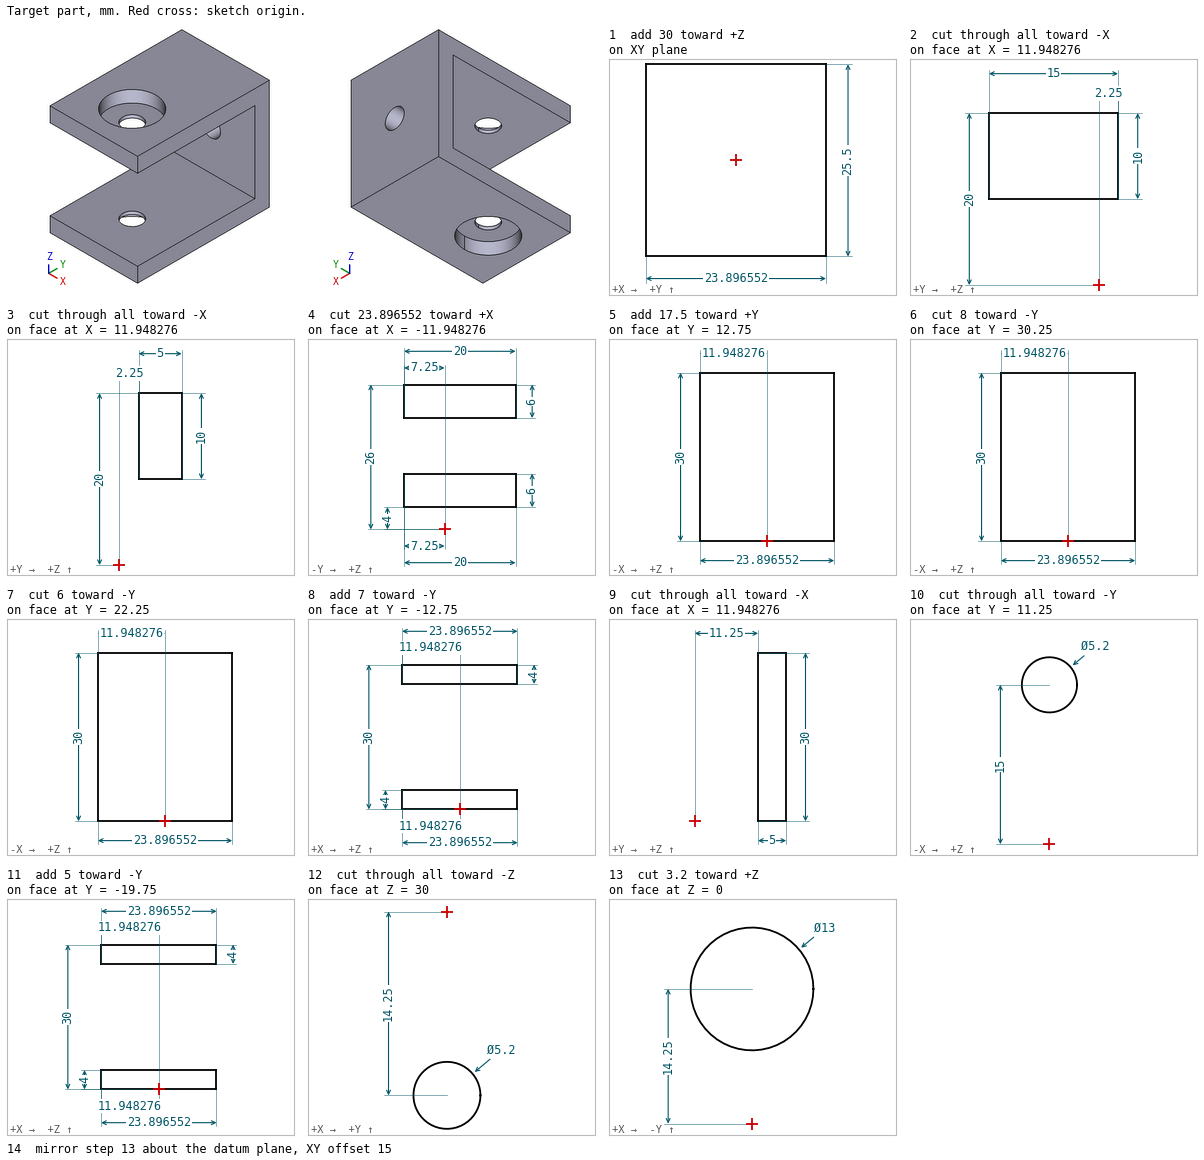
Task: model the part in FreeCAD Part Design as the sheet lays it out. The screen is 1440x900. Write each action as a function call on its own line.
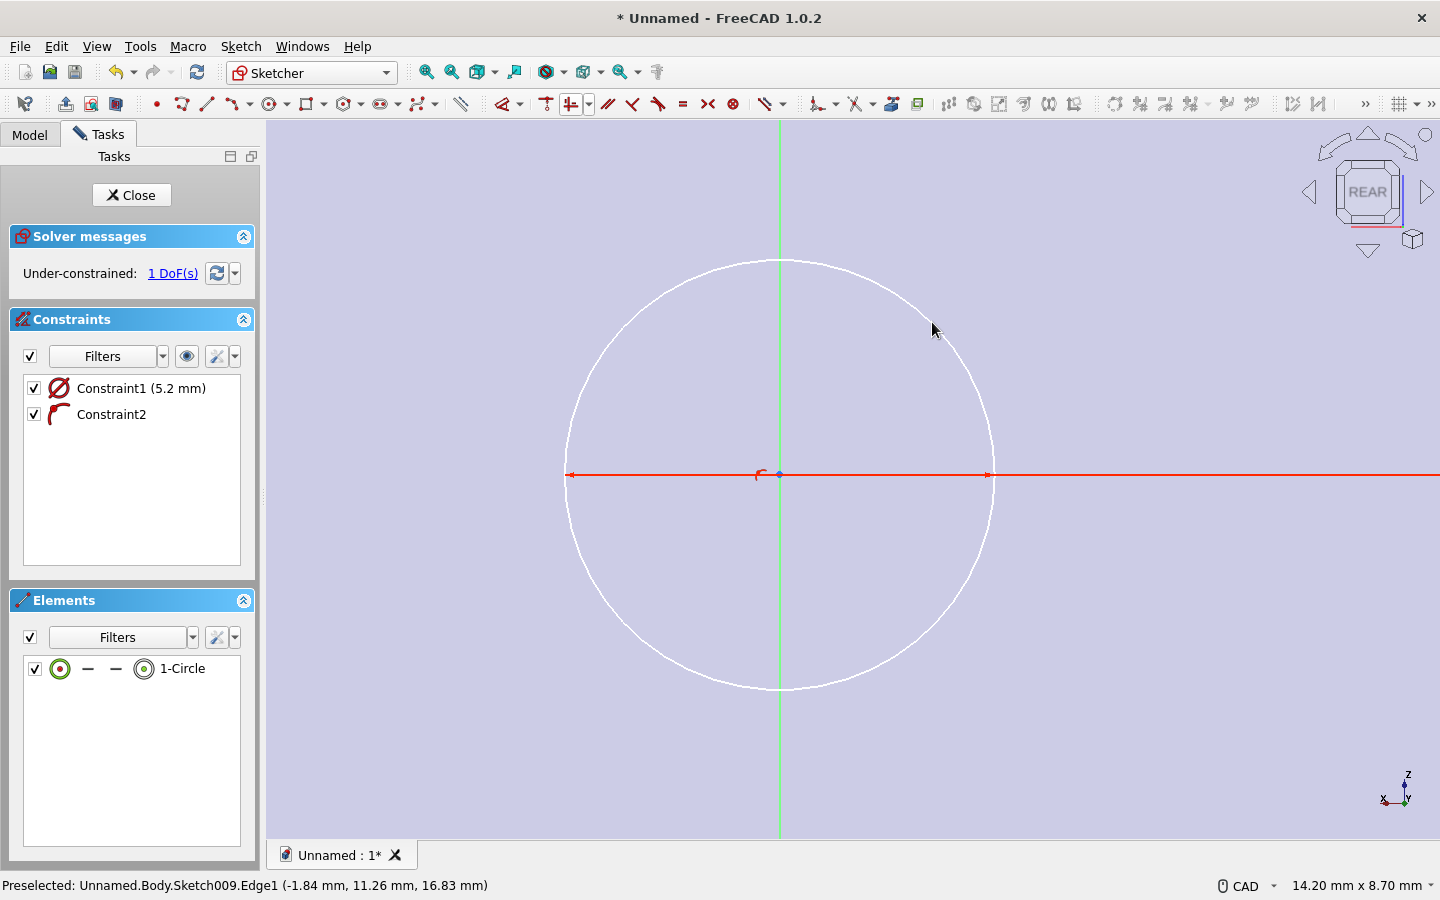
key(d)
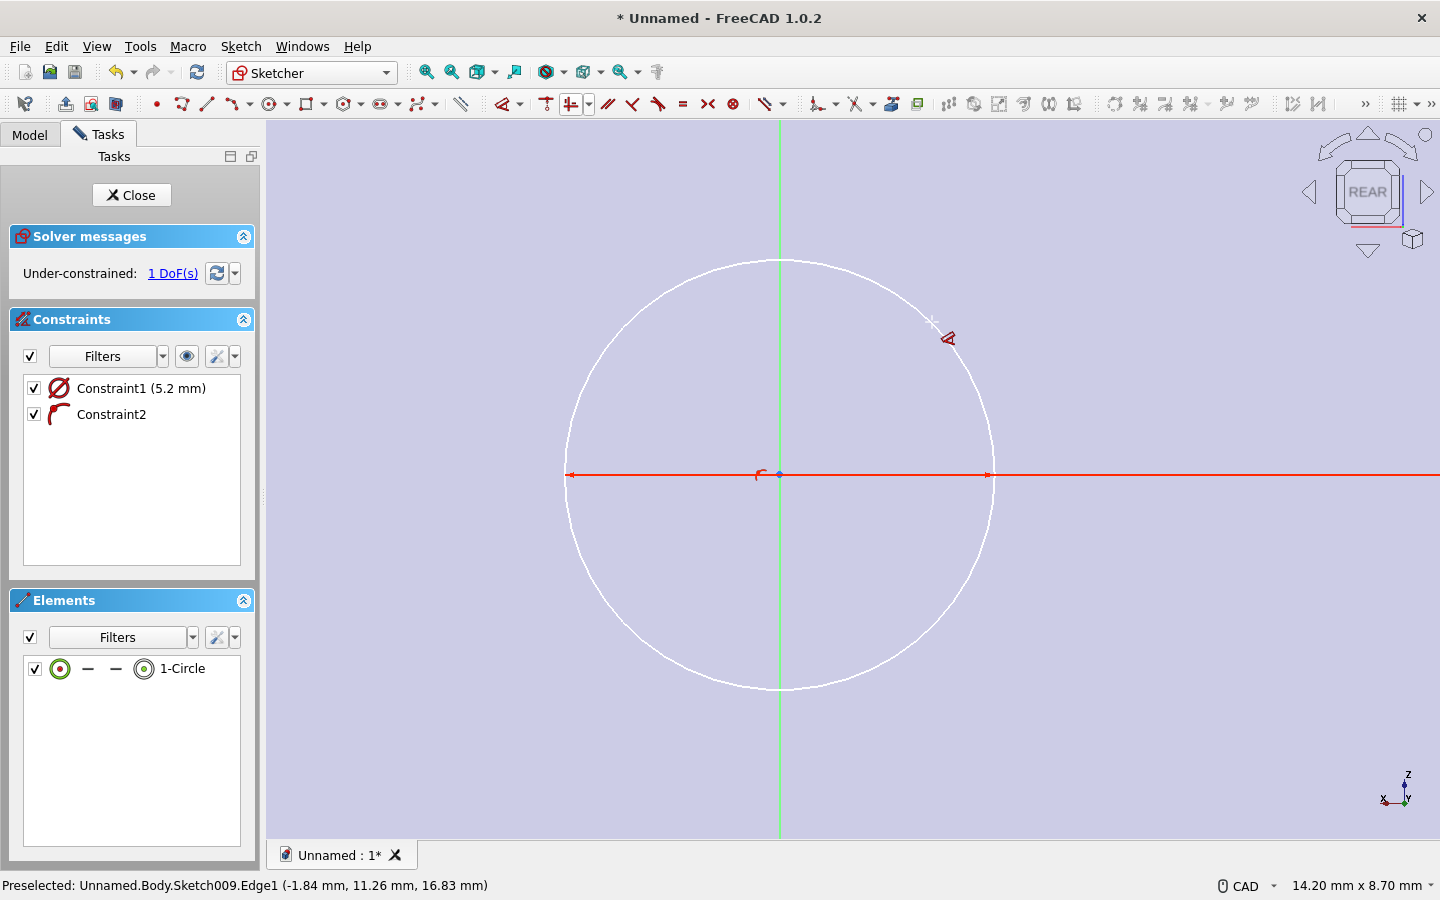
click(780, 475)
click(814, 643)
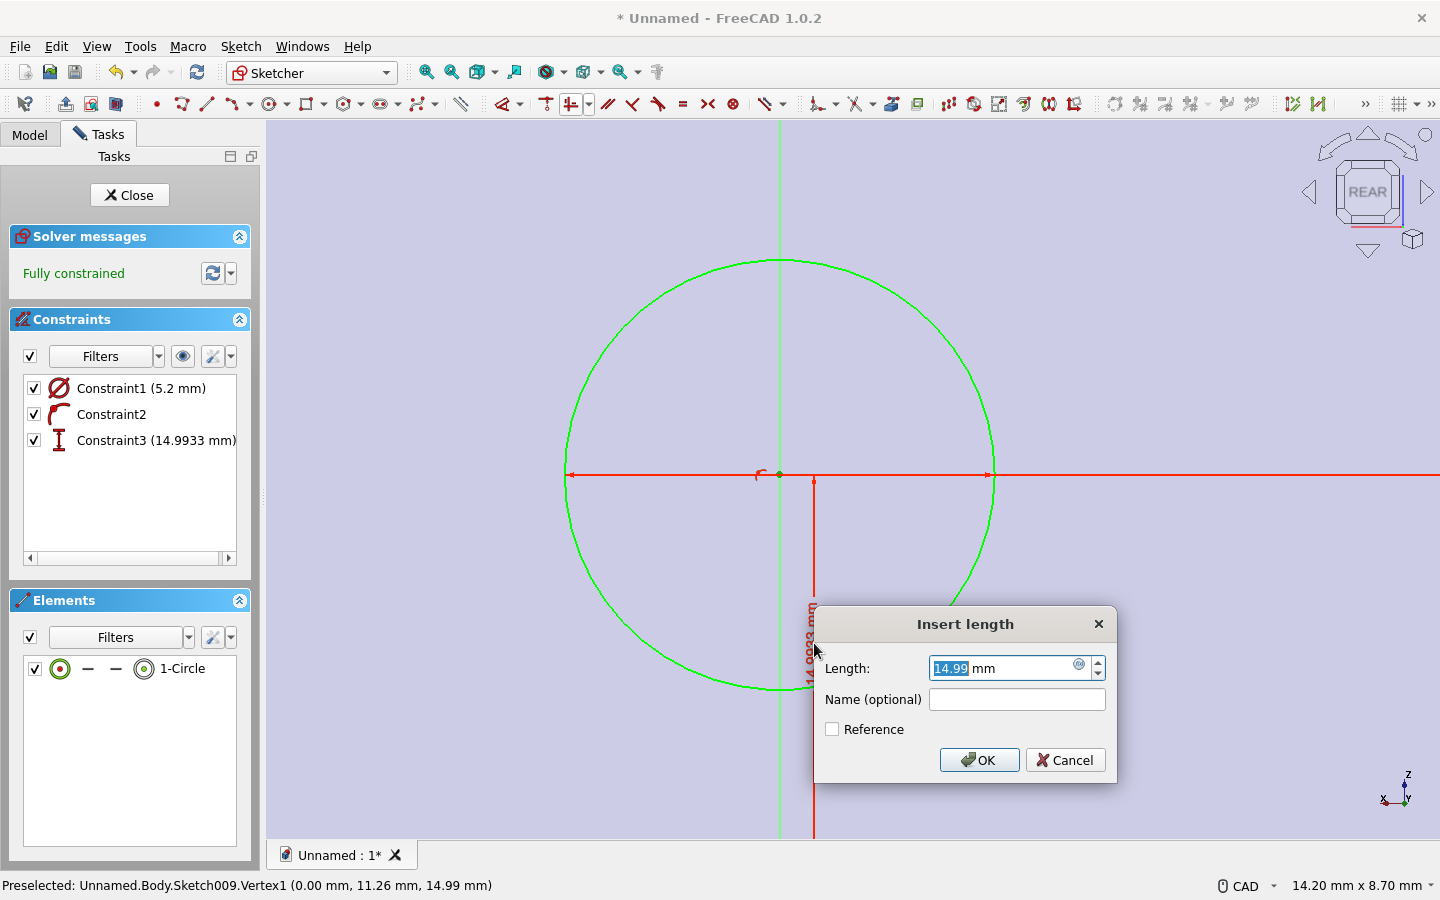
text(15)
key(Return)
key(Escape)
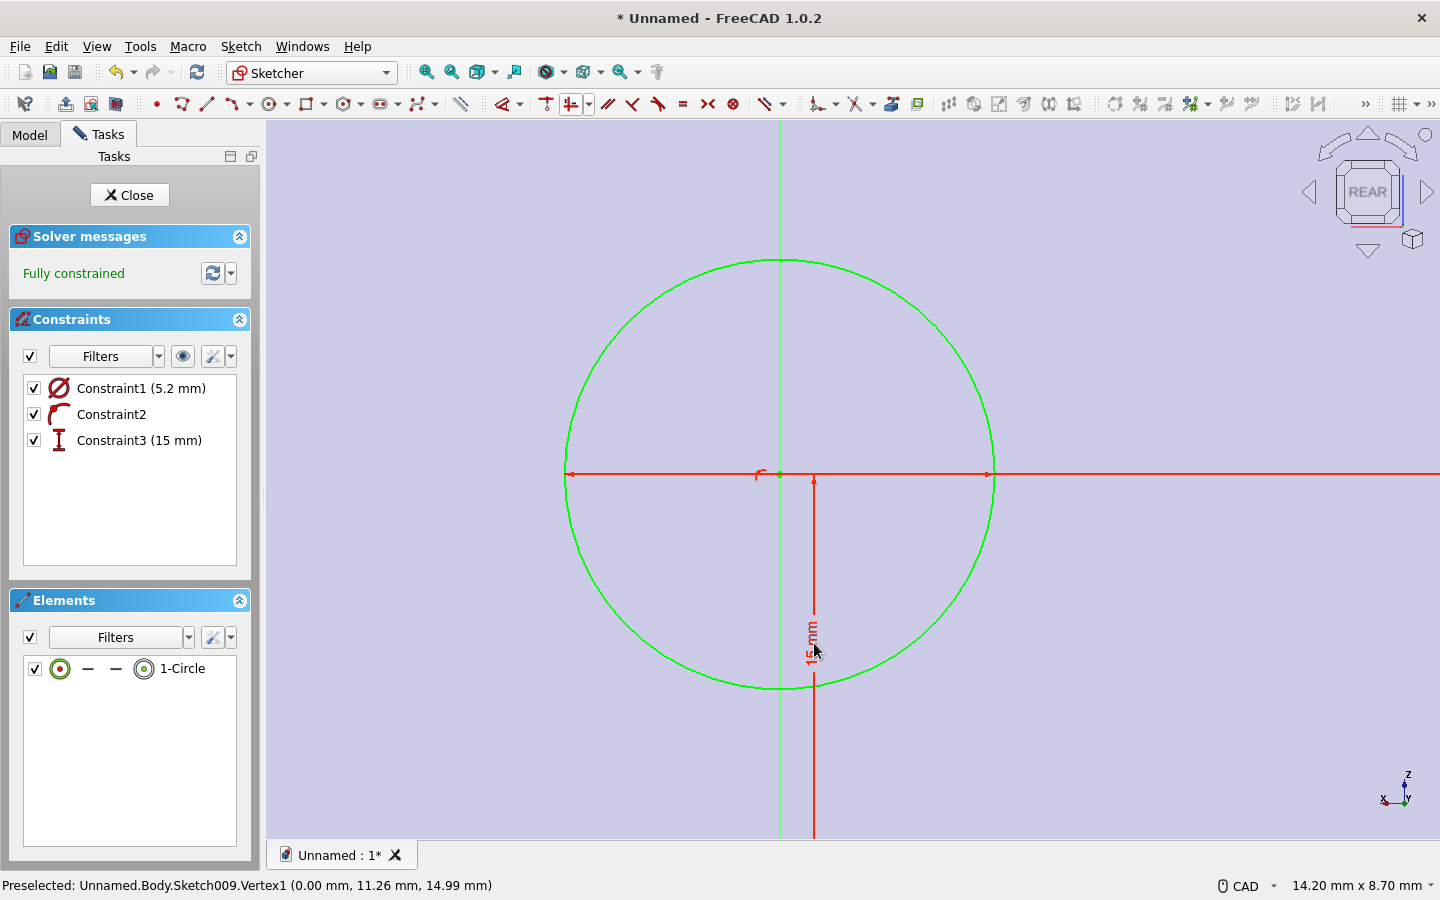
click(130, 195)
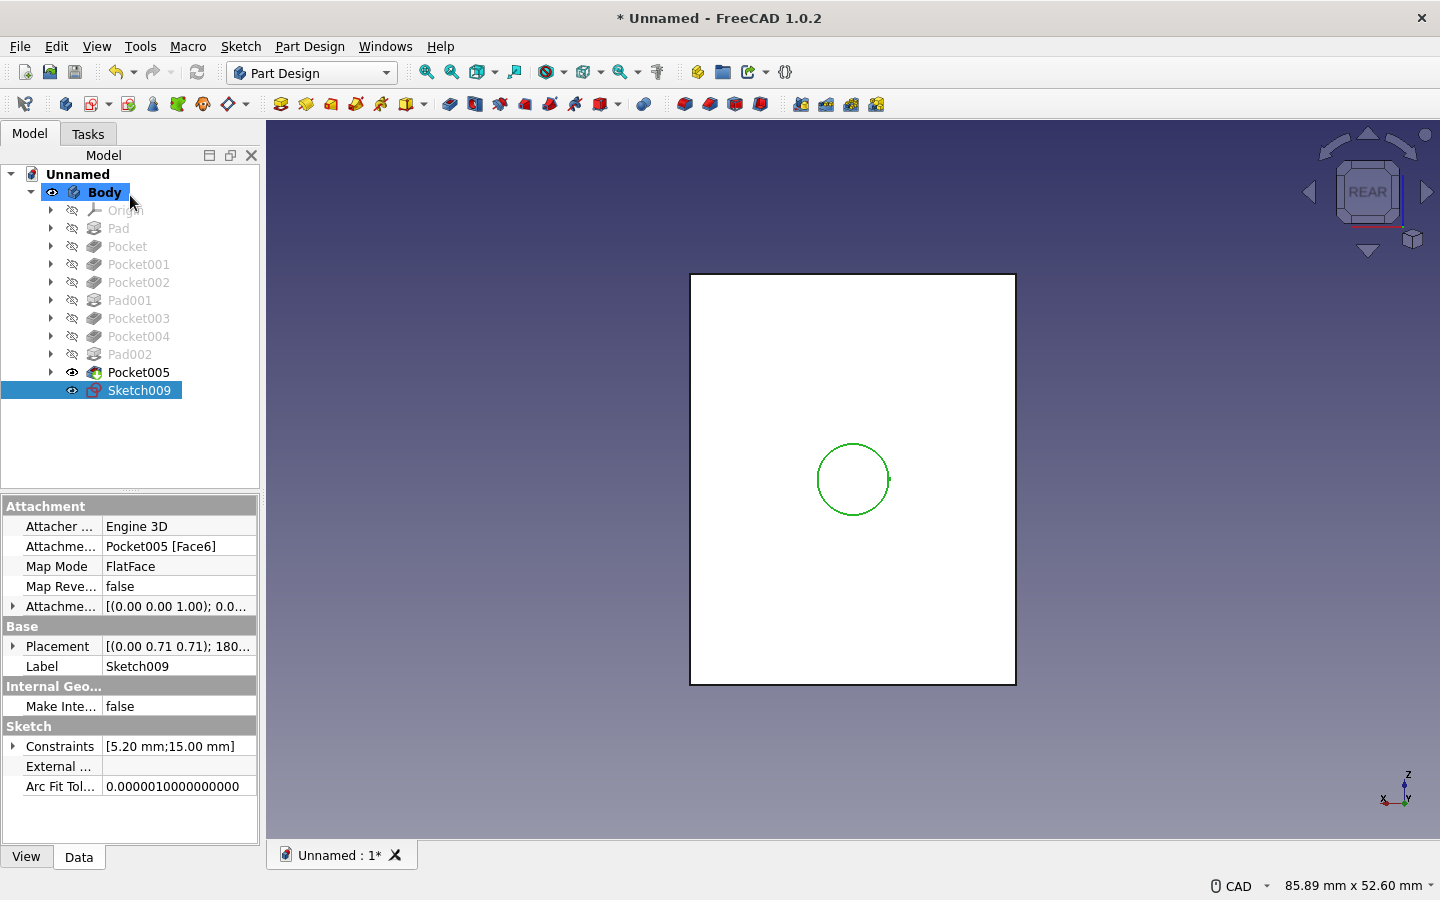
click(450, 104)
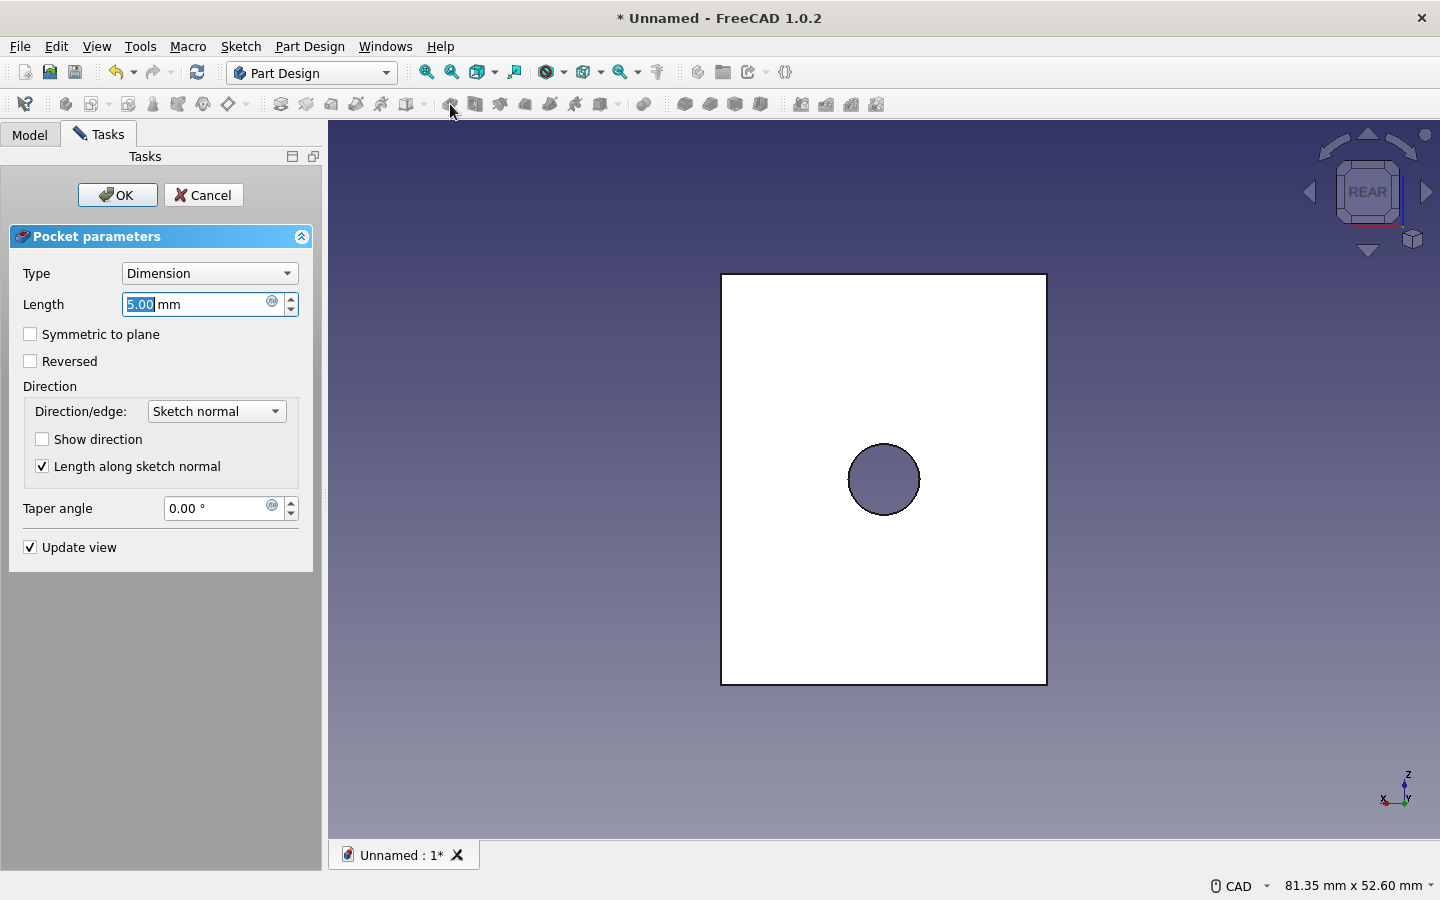
click(210, 274)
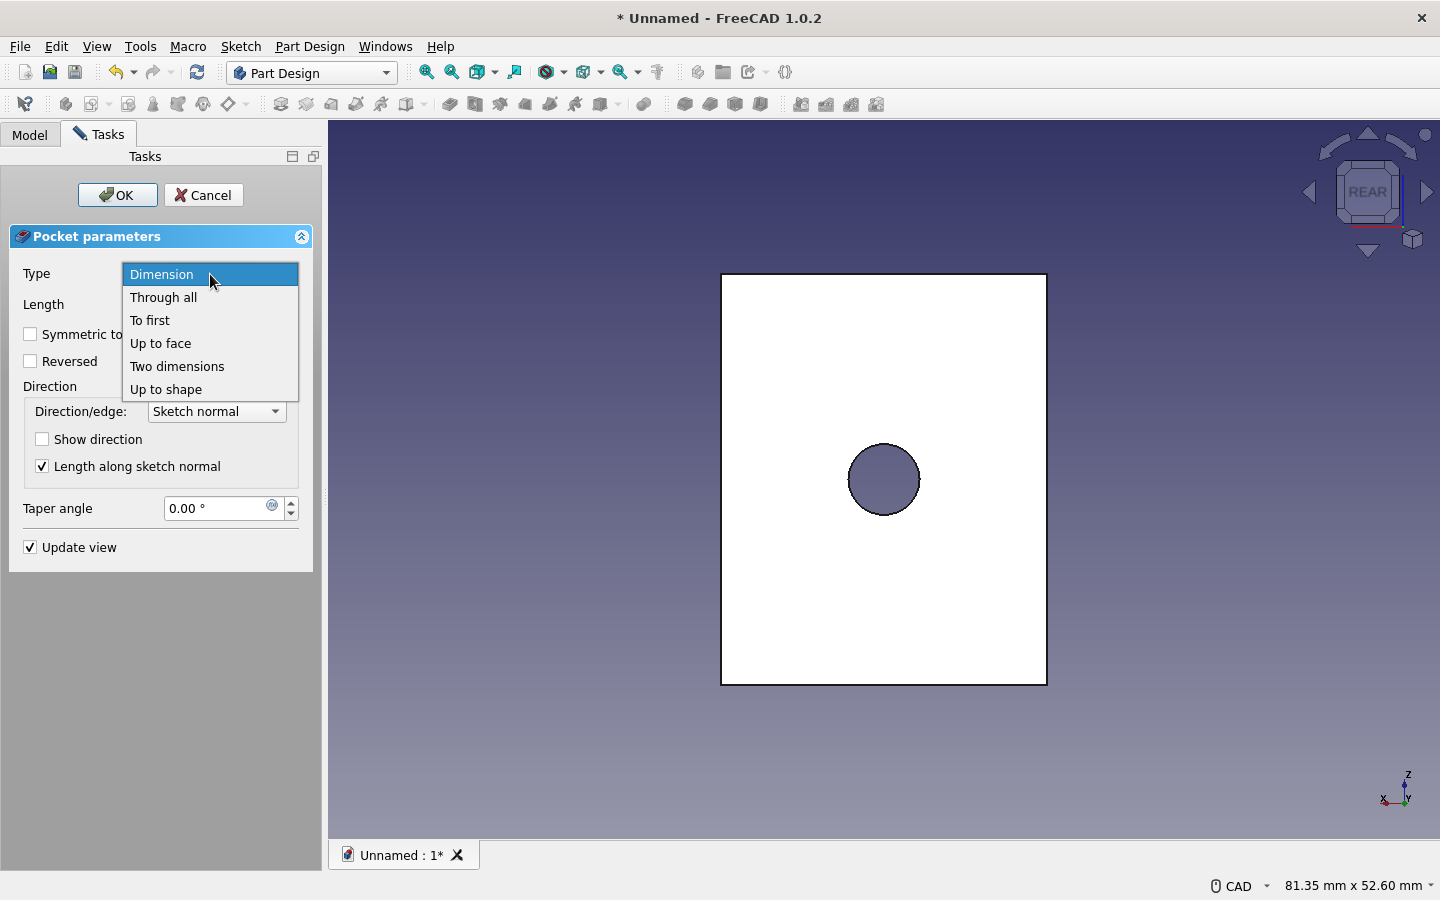
click(208, 298)